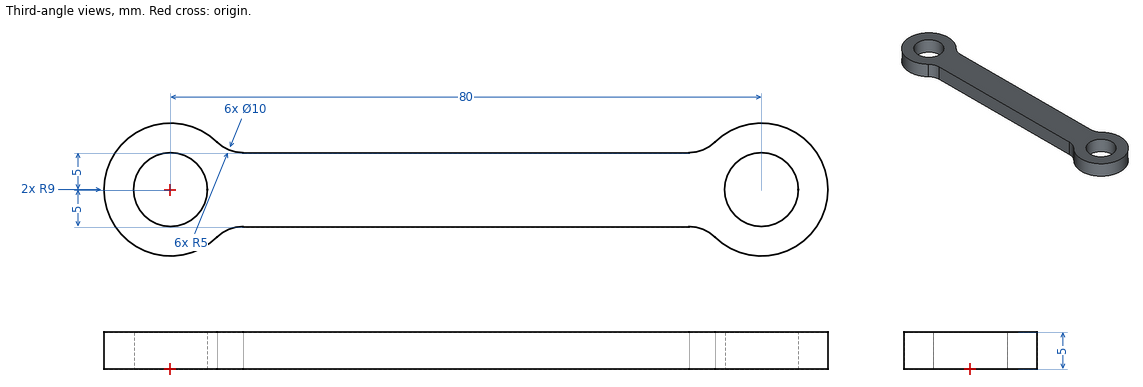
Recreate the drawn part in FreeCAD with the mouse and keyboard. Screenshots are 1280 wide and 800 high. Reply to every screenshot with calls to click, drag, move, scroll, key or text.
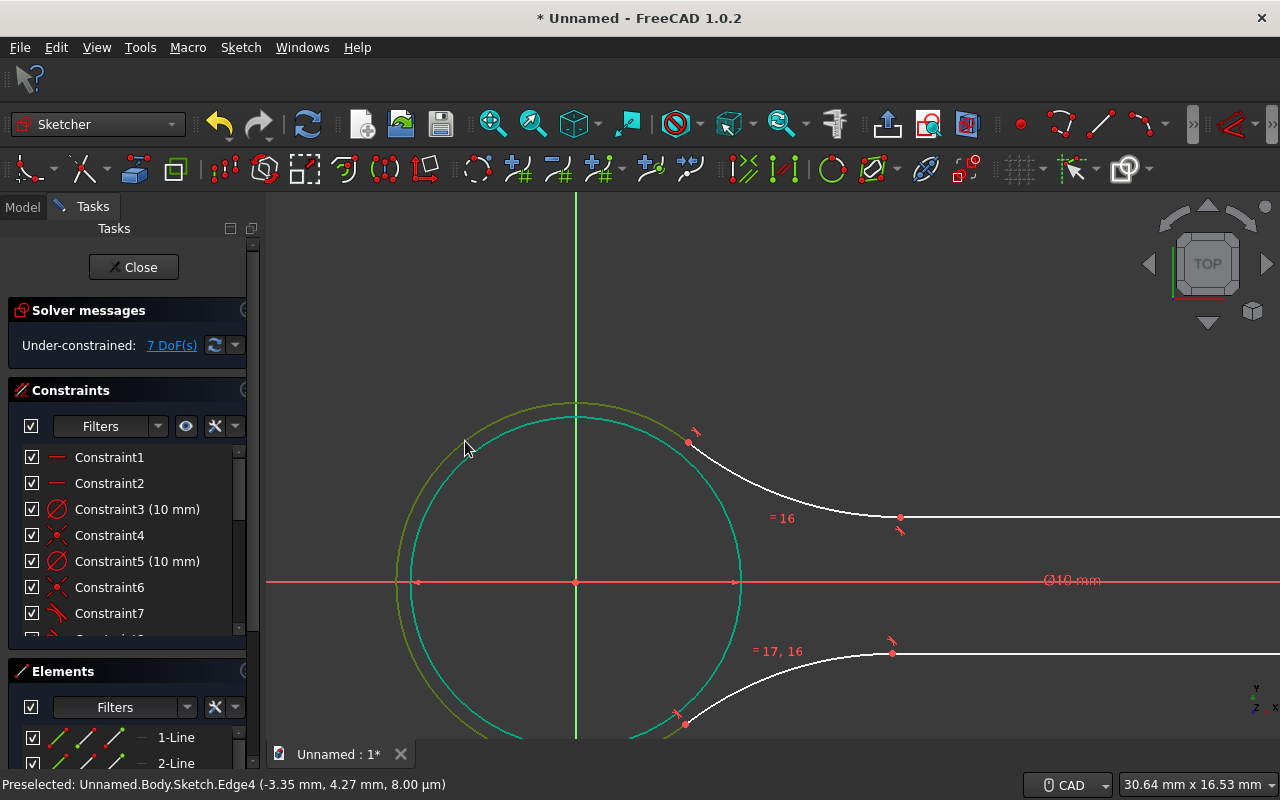
scroll(468, 442, down, 9)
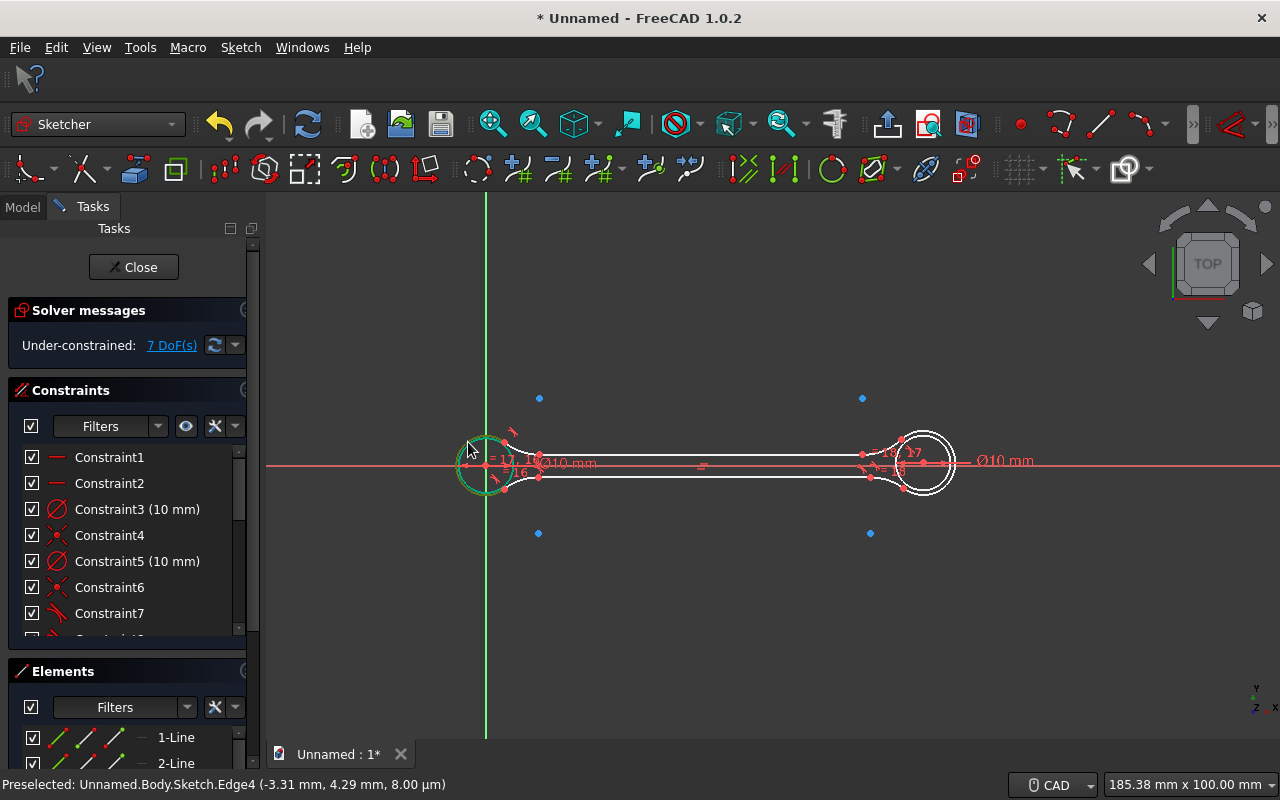
scroll(944, 487, up, 6)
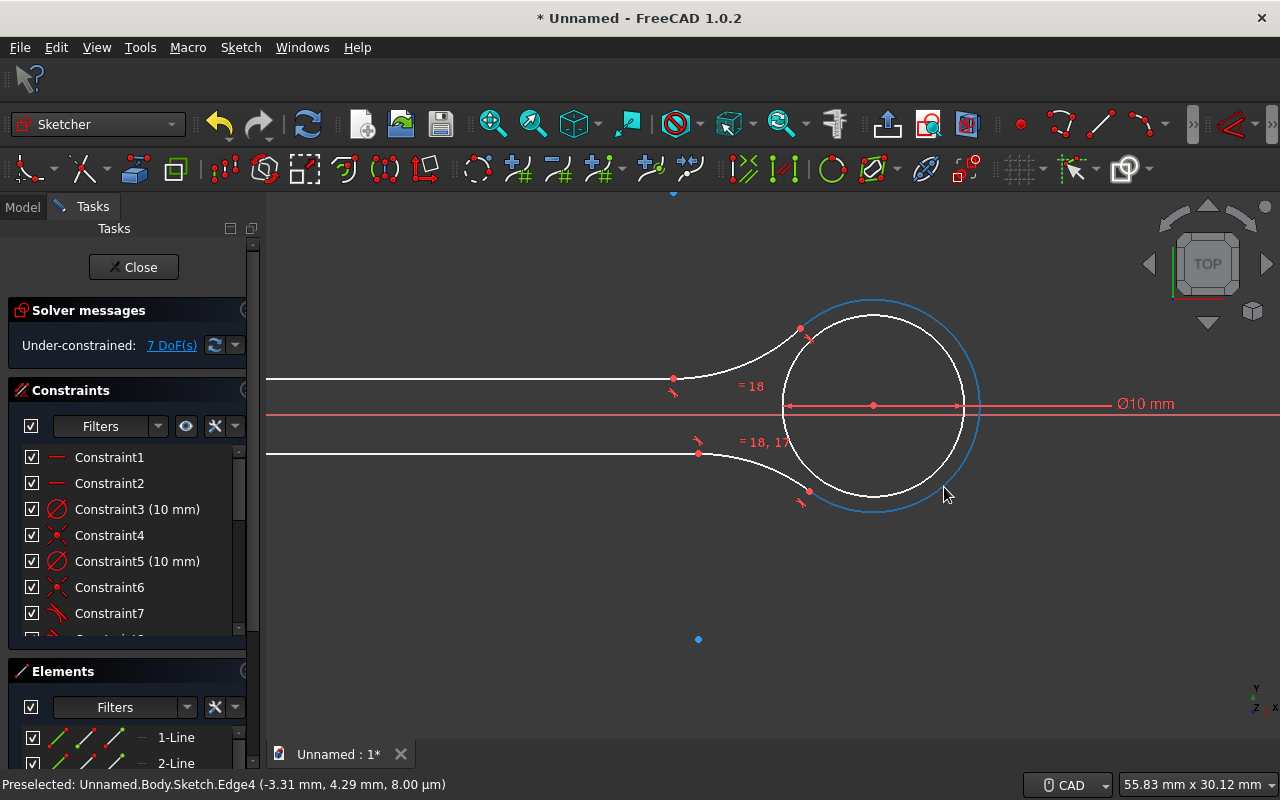
click(943, 486)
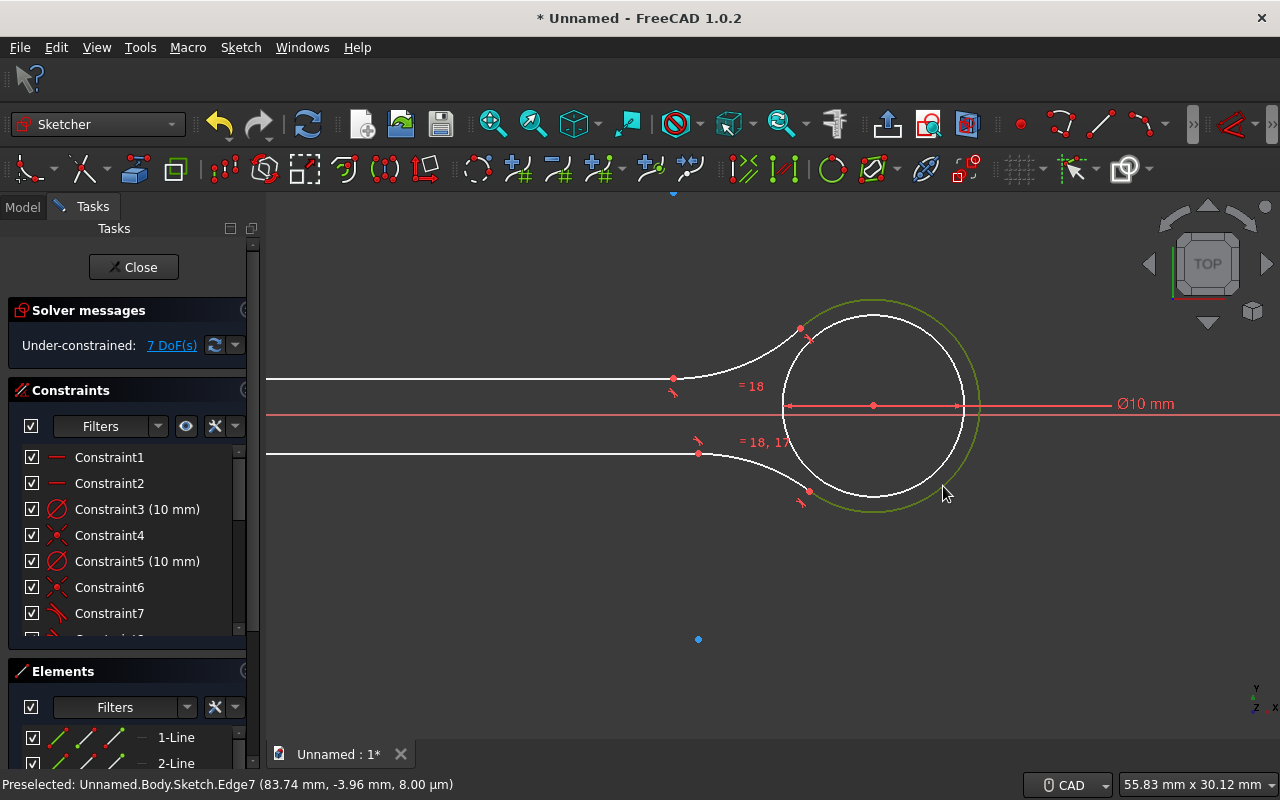
key(e)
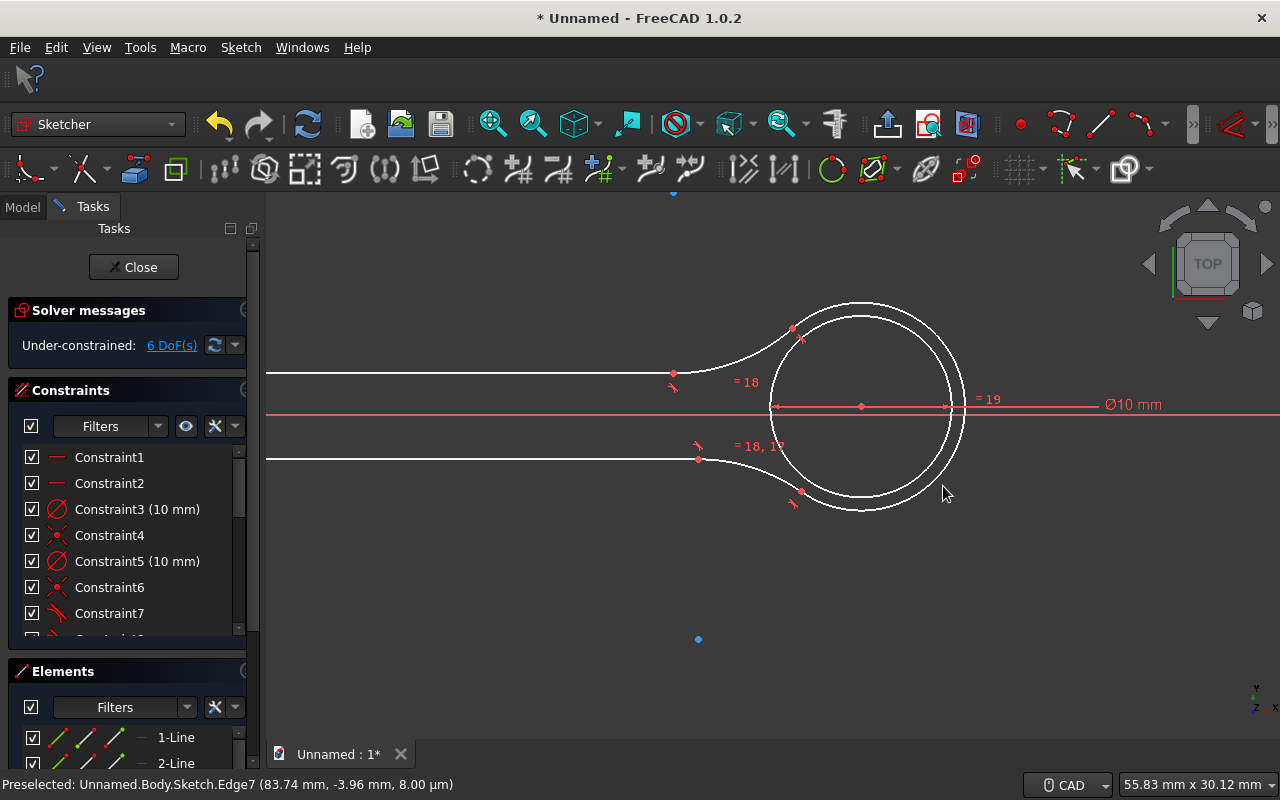
scroll(944, 487, down, 6)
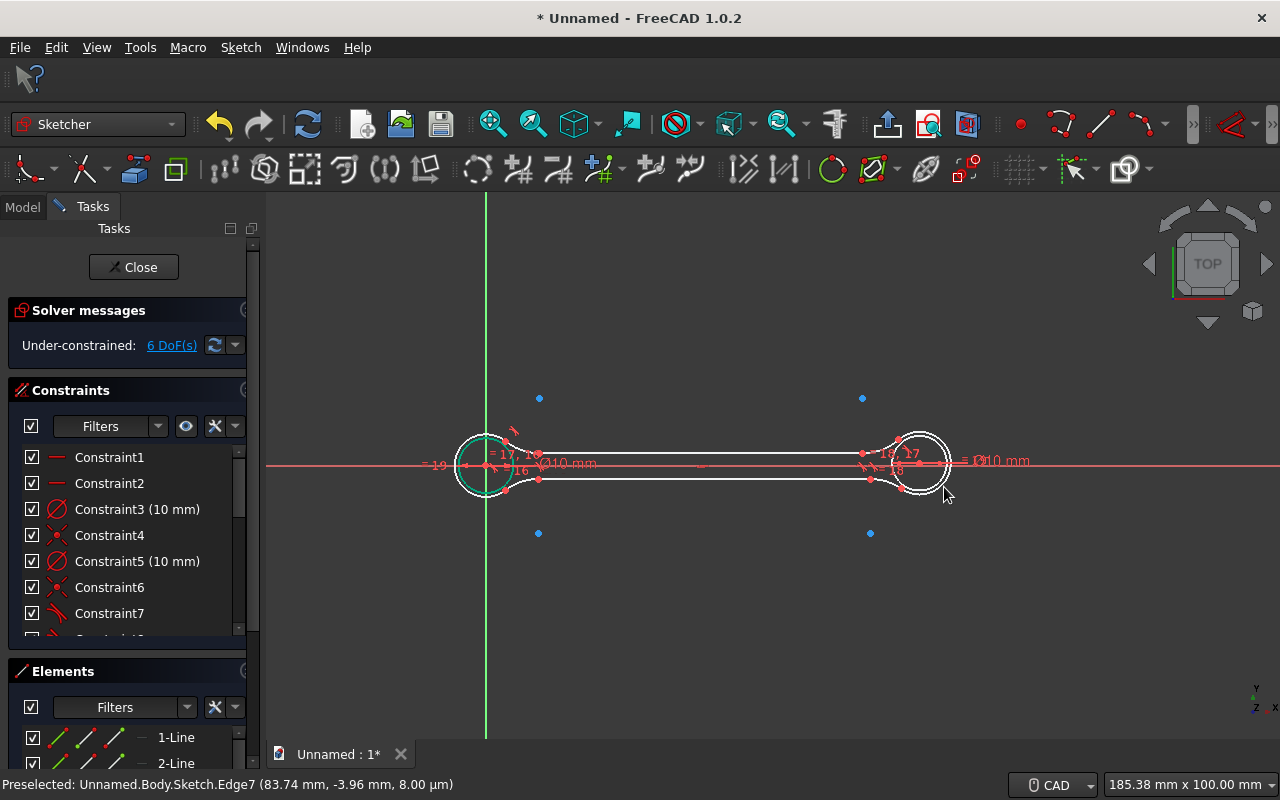
click(919, 463)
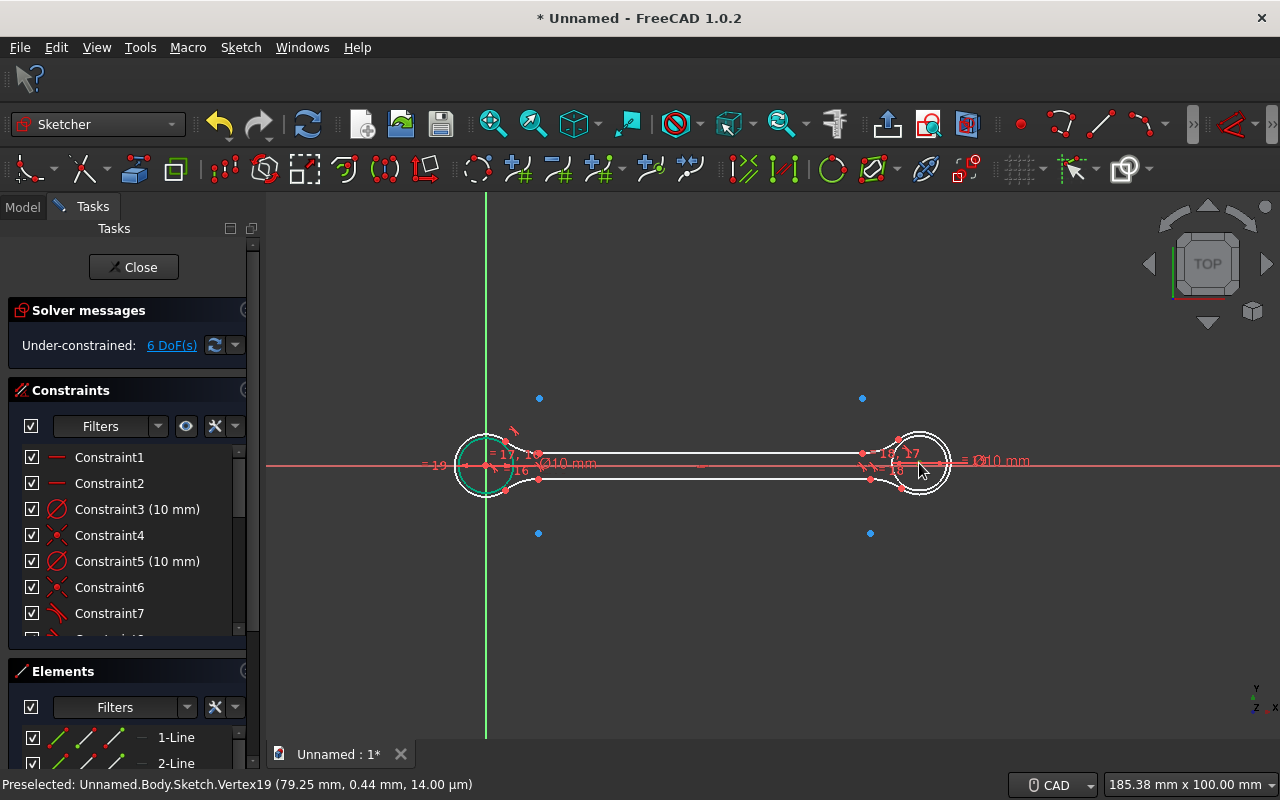
click(353, 466)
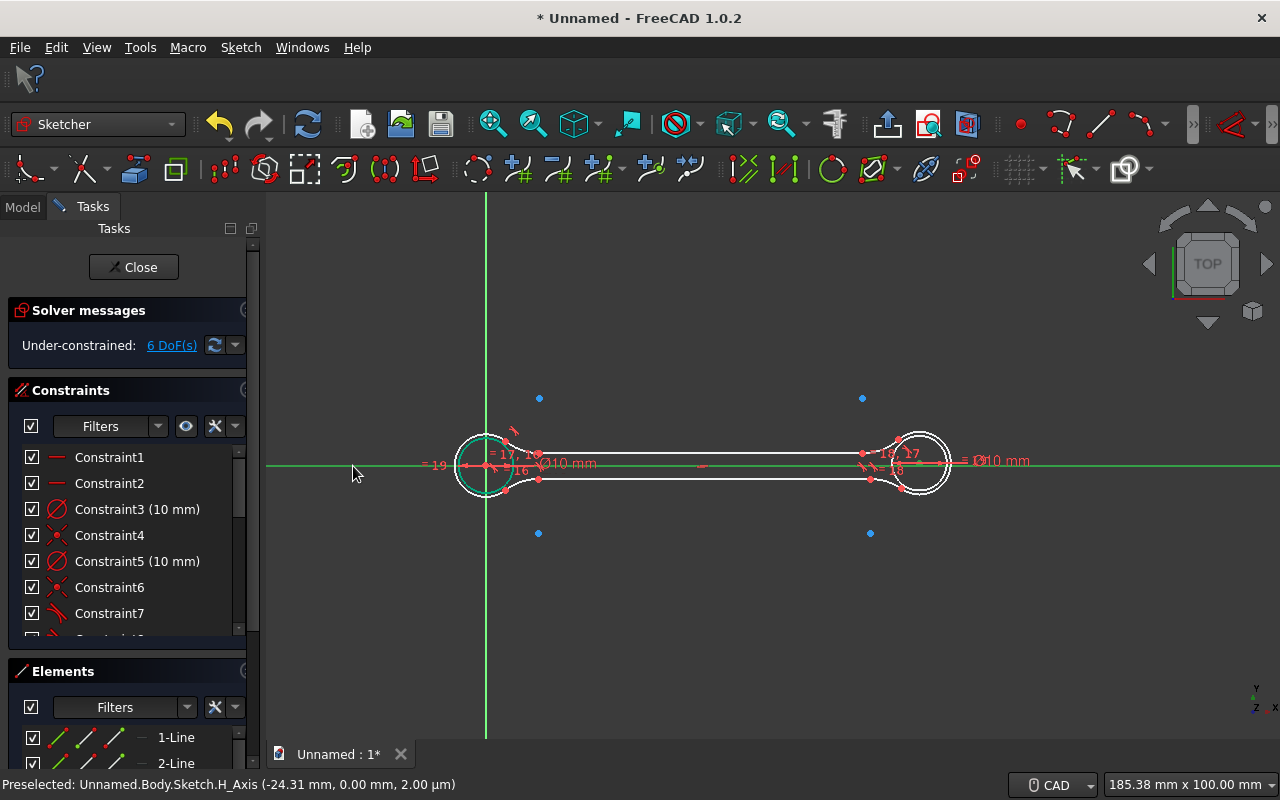
key(c)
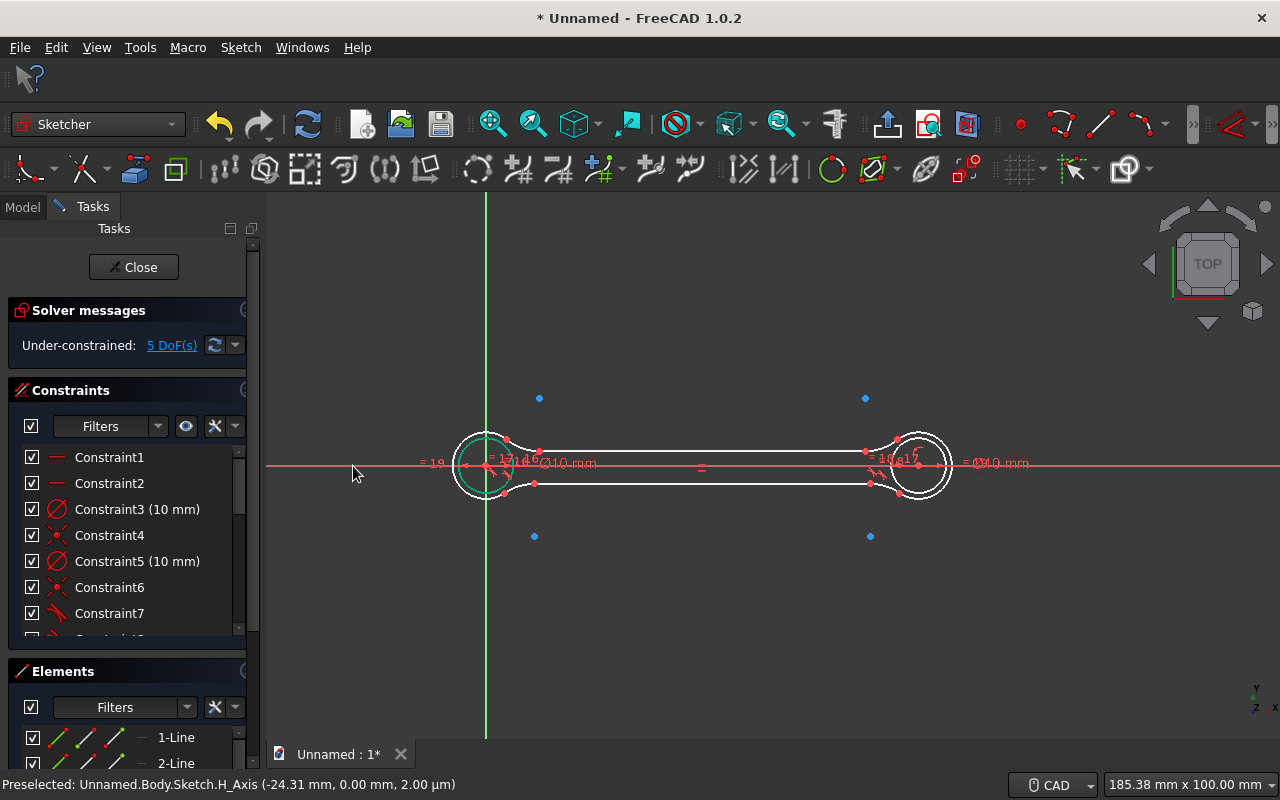
key(d)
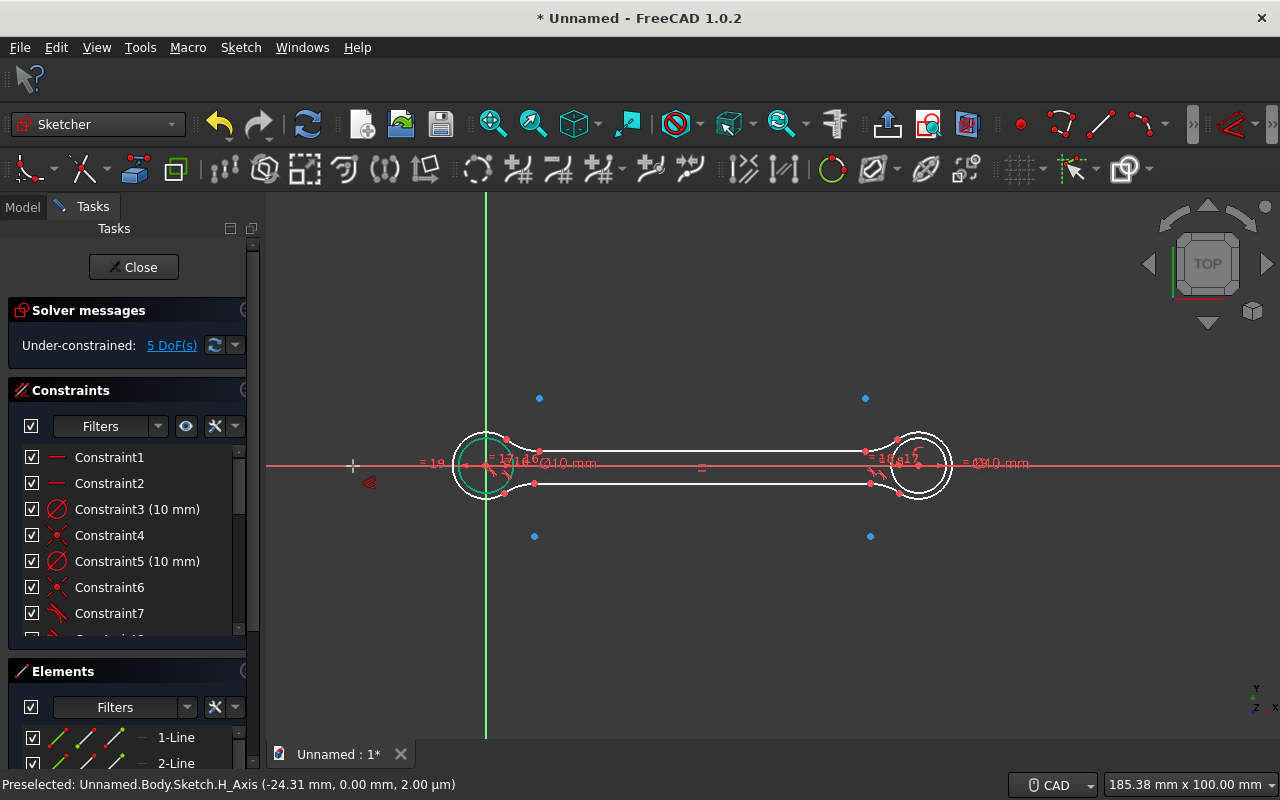
scroll(529, 450, up, 2)